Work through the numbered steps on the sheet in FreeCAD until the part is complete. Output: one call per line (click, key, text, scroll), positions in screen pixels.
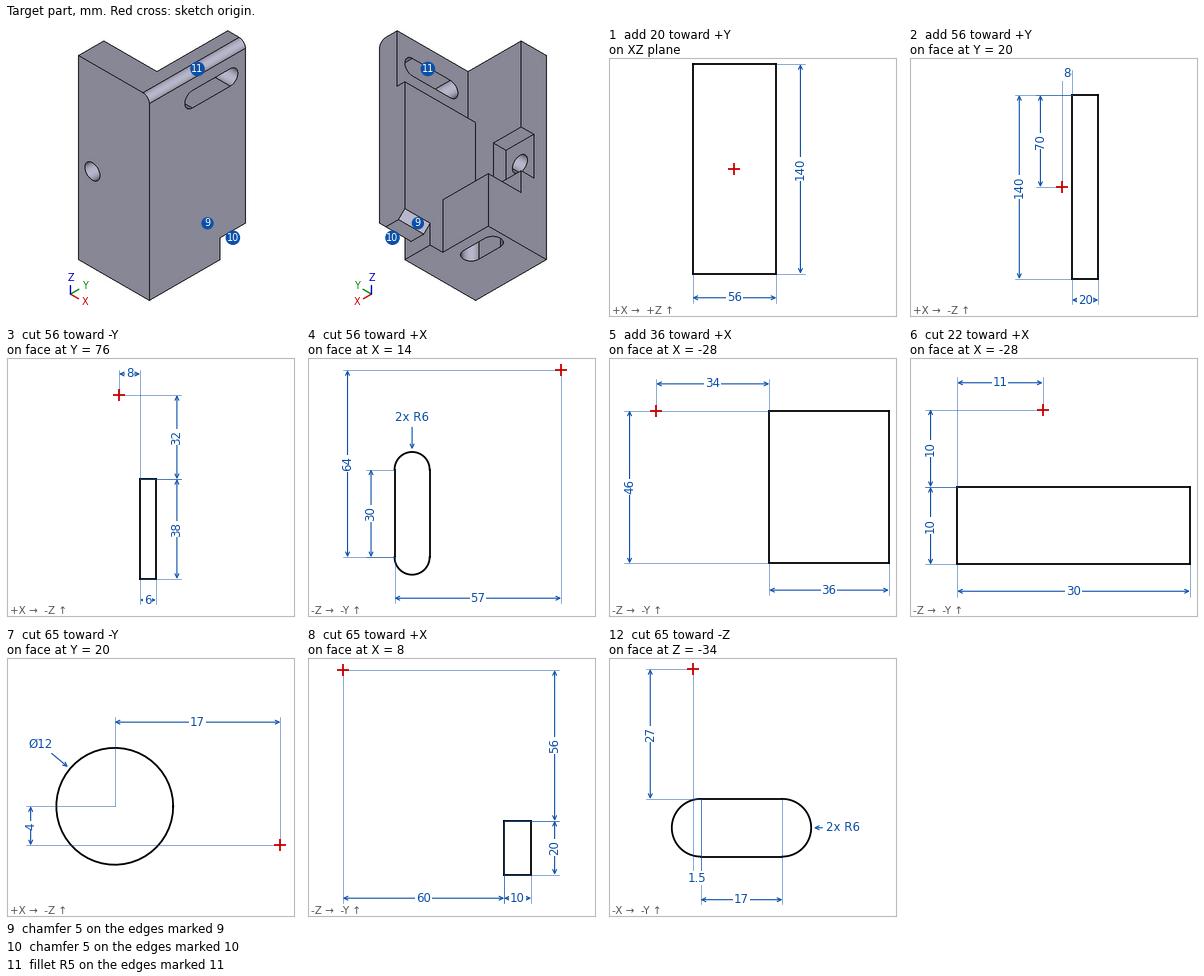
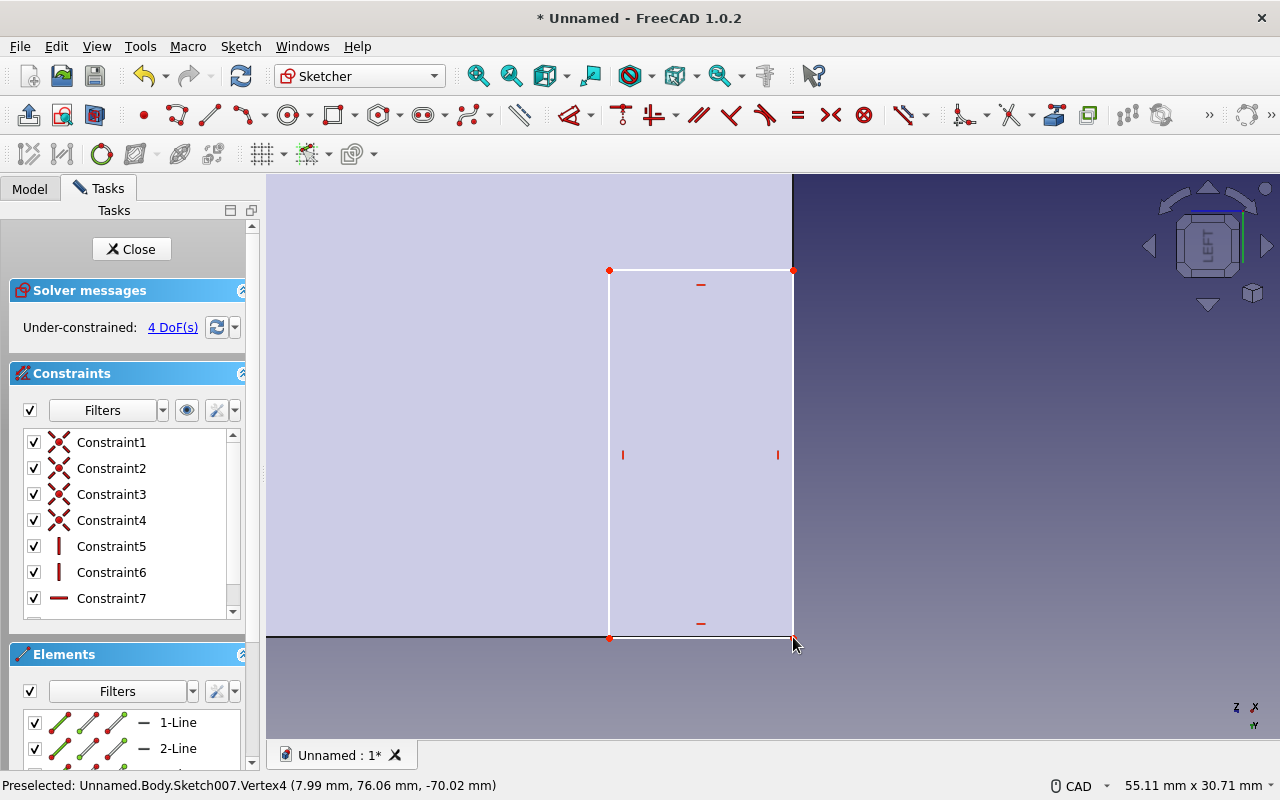
click(568, 116)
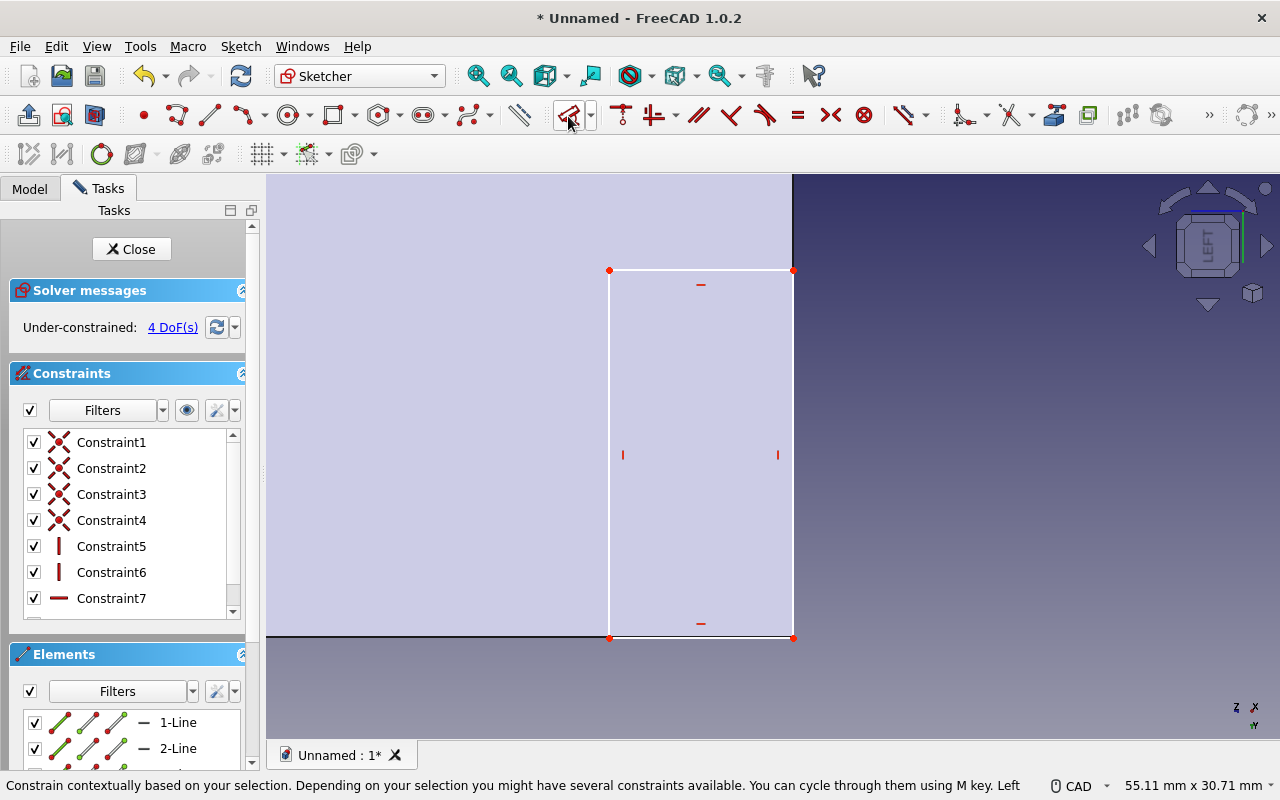
click(609, 380)
click(575, 454)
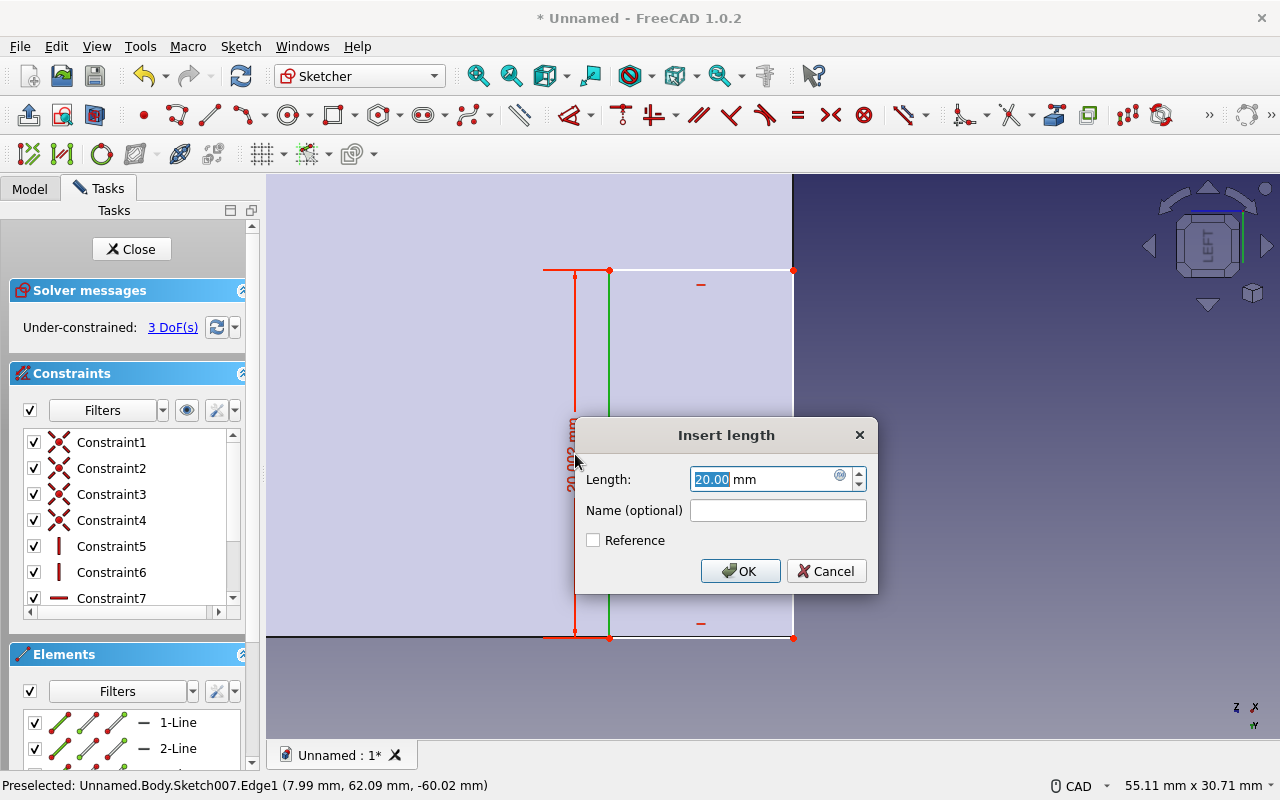
text(20)
key(Return)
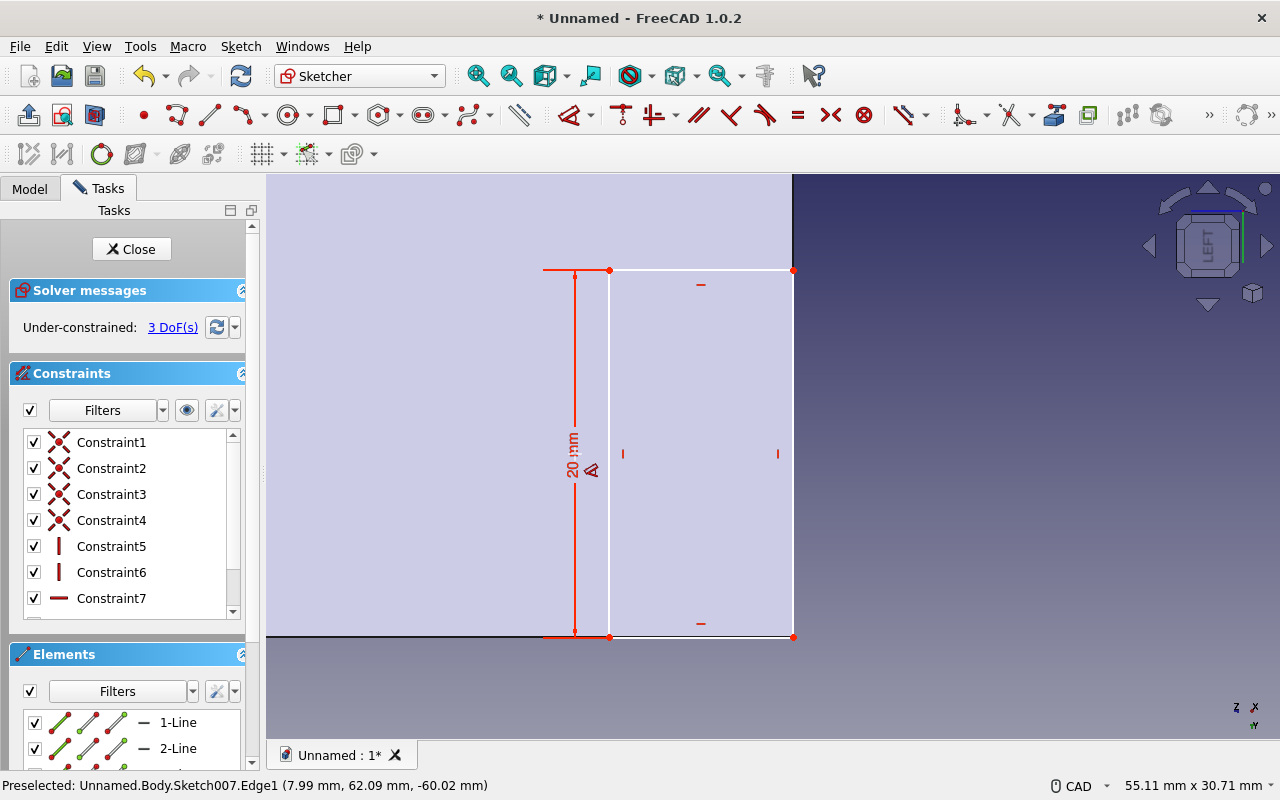
click(664, 638)
click(701, 672)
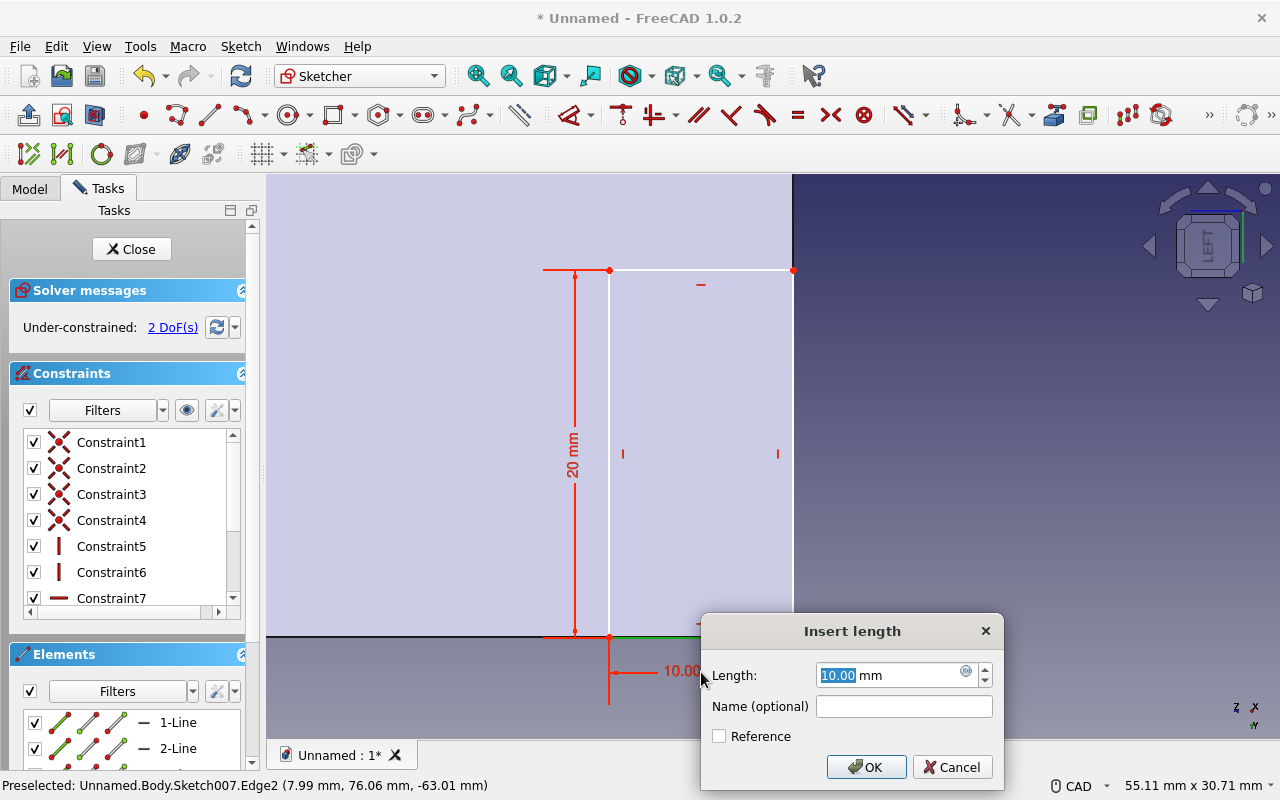
text(10)
key(Return)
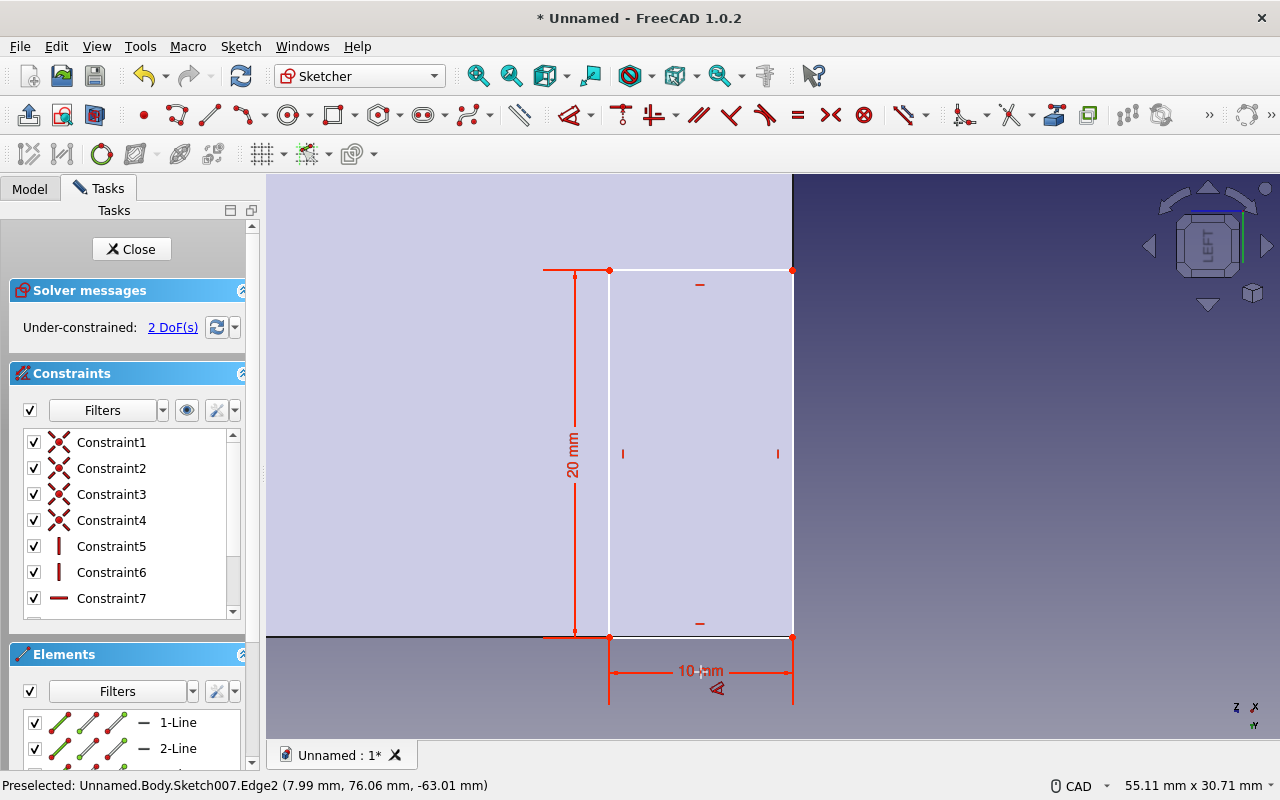
click(609, 270)
click(452, 304)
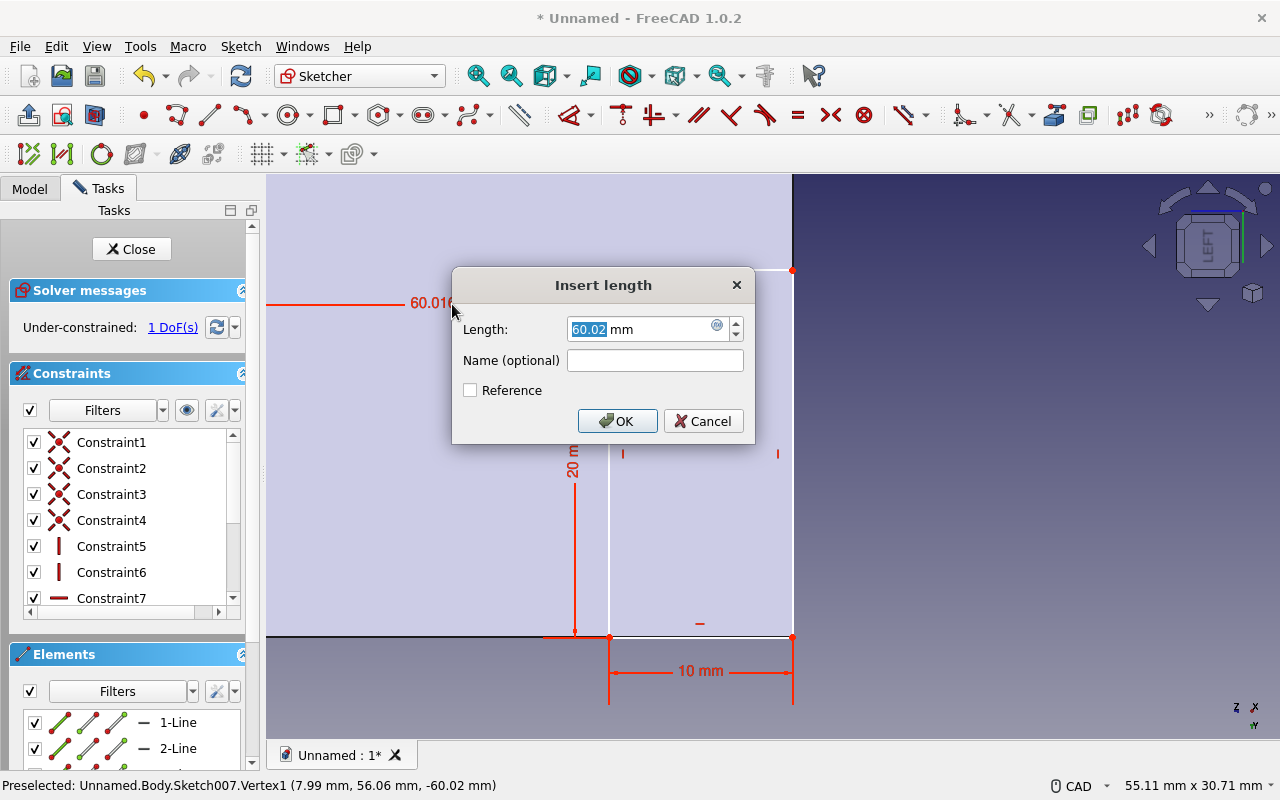
text(60)
key(Return)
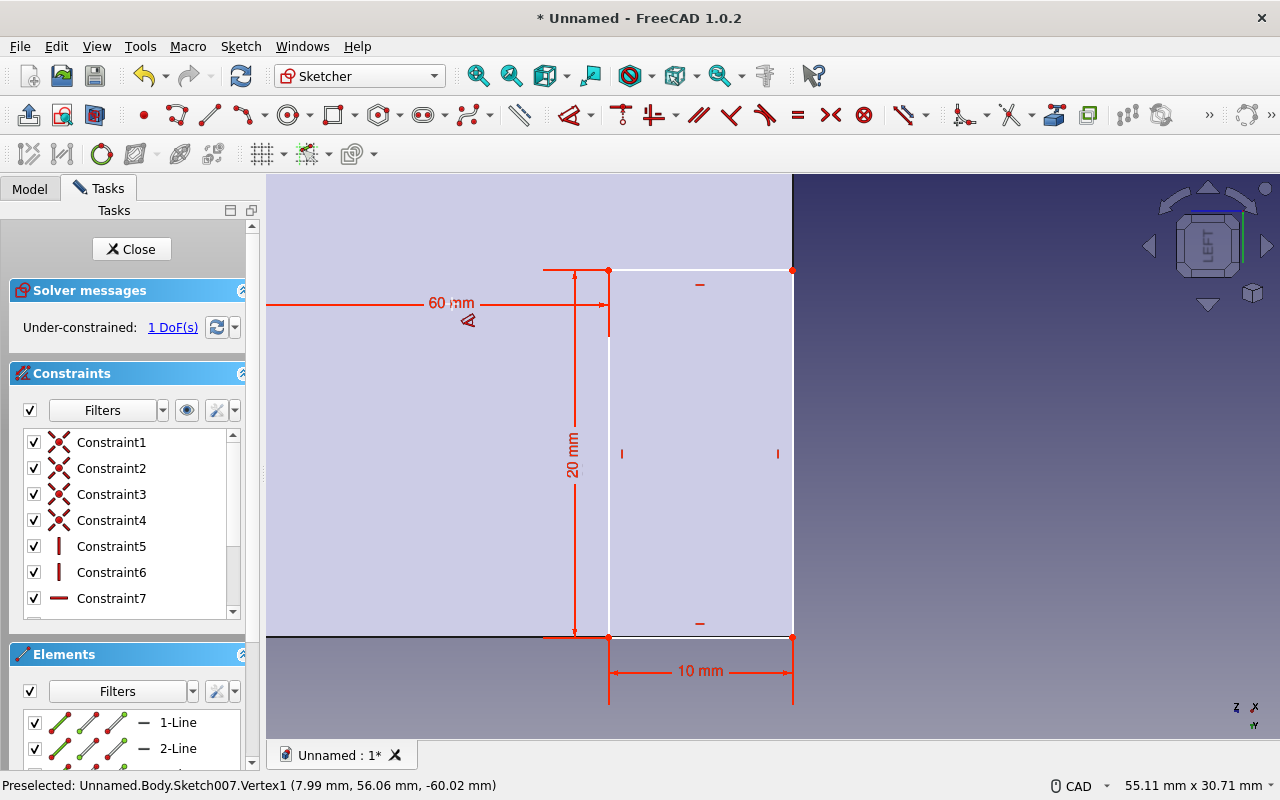
click(609, 270)
click(643, 236)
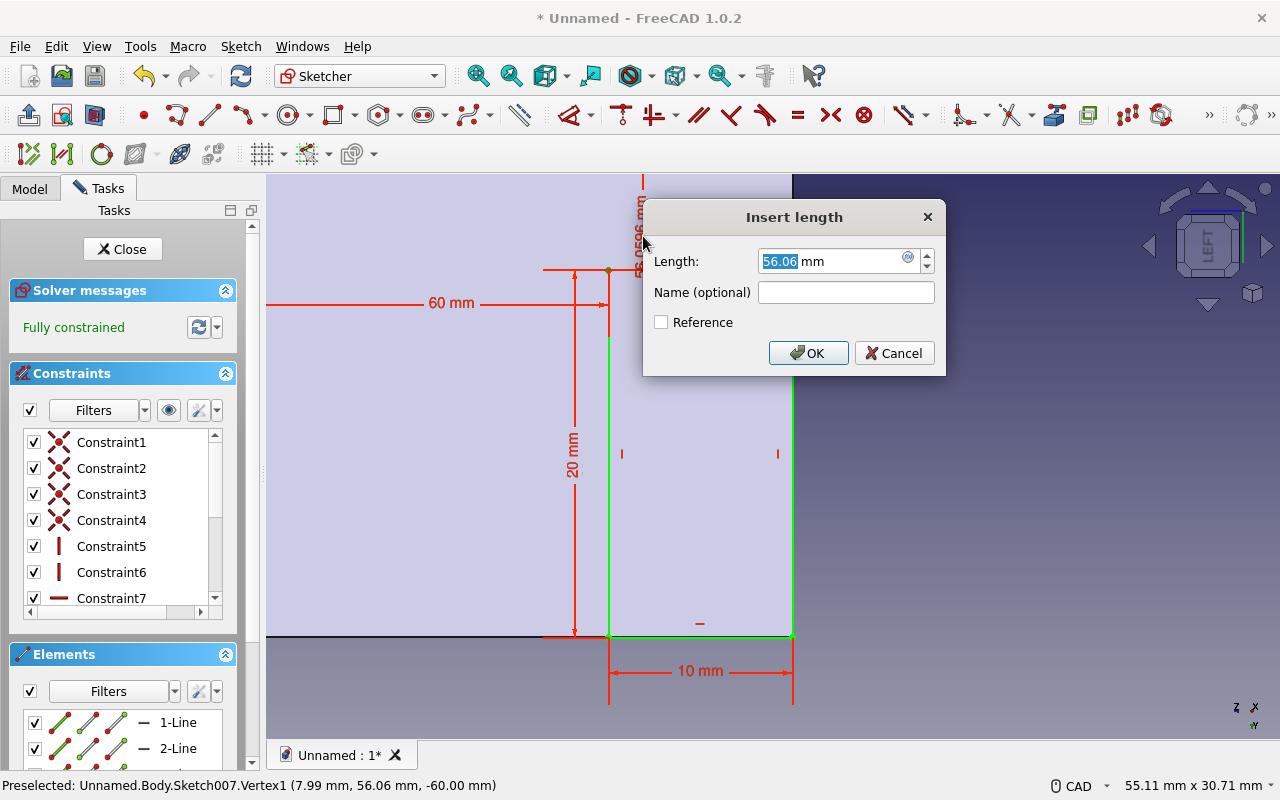
text(56)
key(Return)
key(Escape)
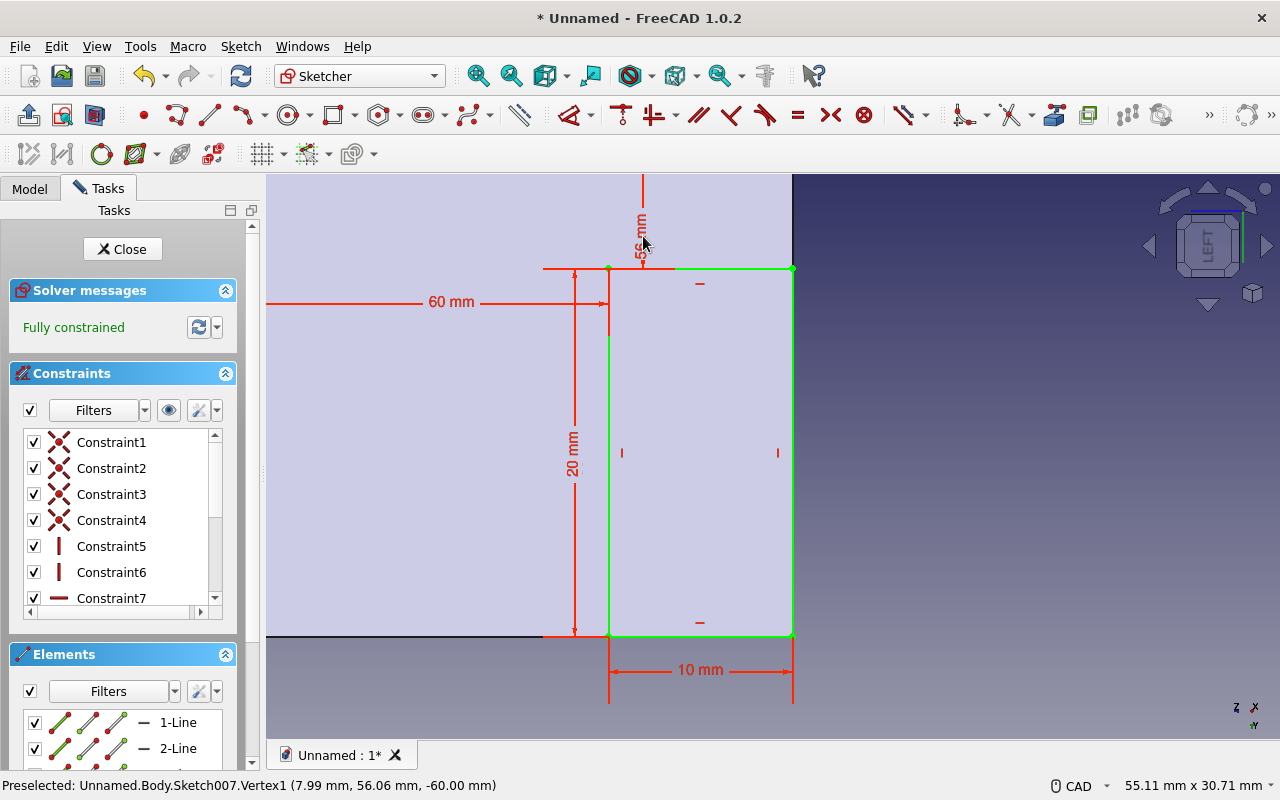
click(123, 249)